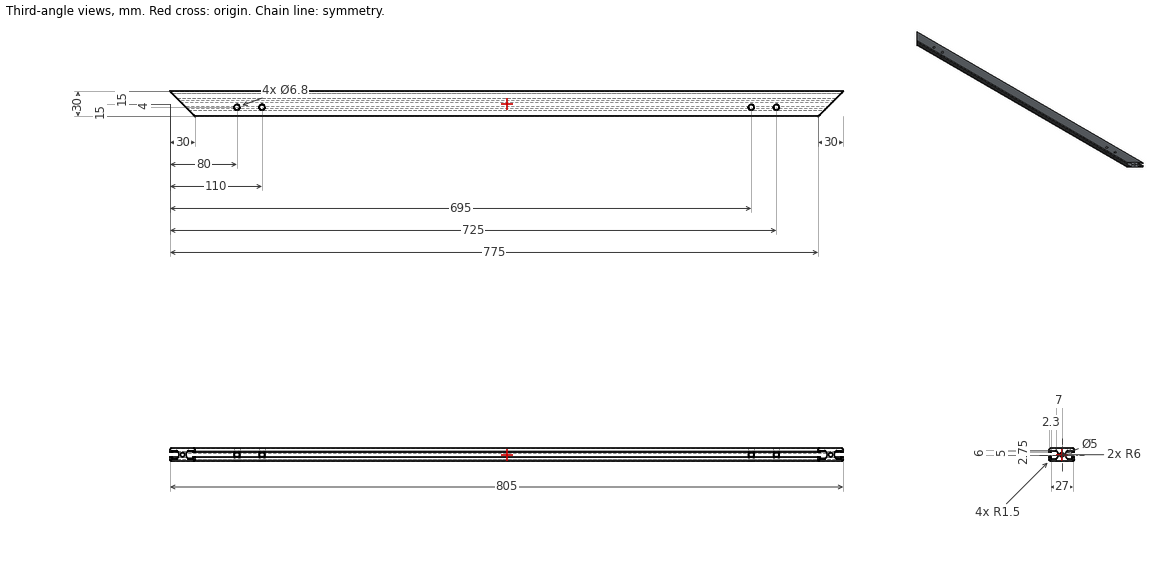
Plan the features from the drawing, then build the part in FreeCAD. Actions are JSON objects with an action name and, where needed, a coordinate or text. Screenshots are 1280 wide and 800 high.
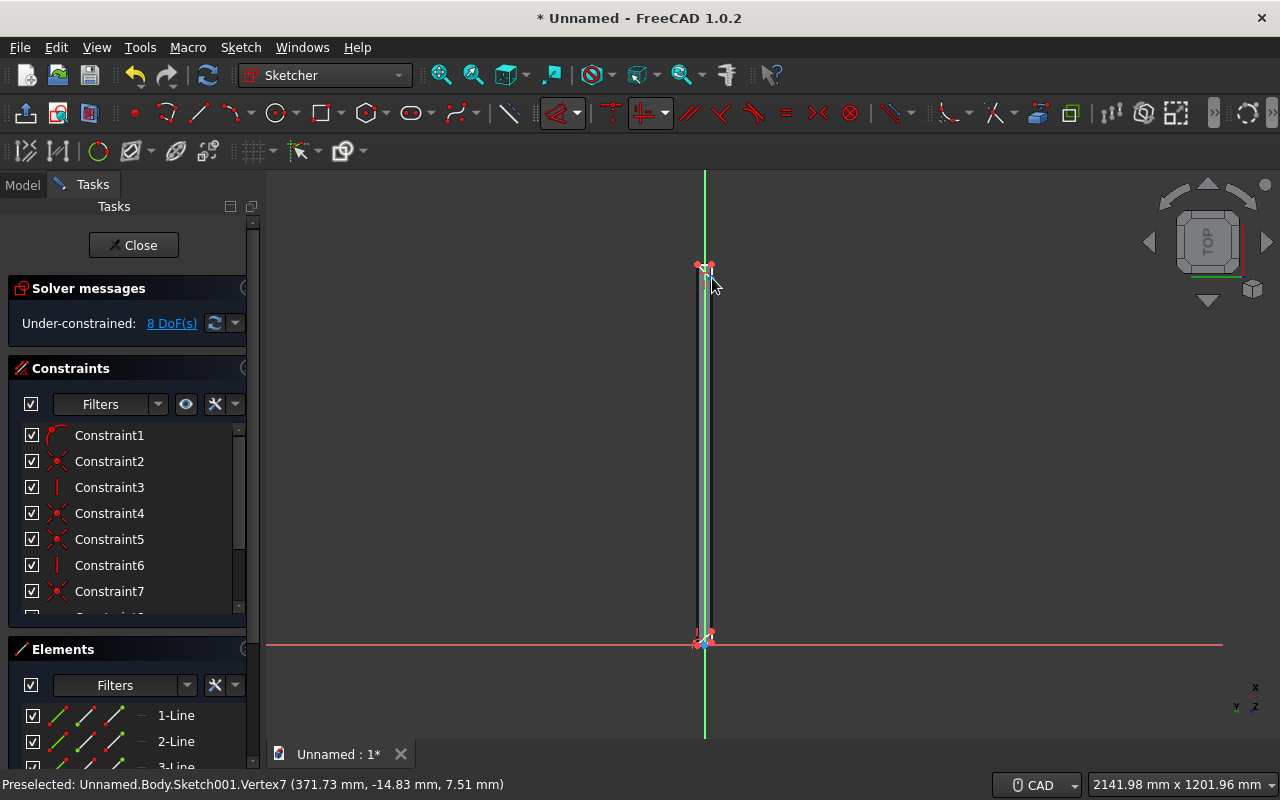
{"action": "scroll", "coordinate": [704, 644], "scroll_direction": "up", "scroll_amount": 7}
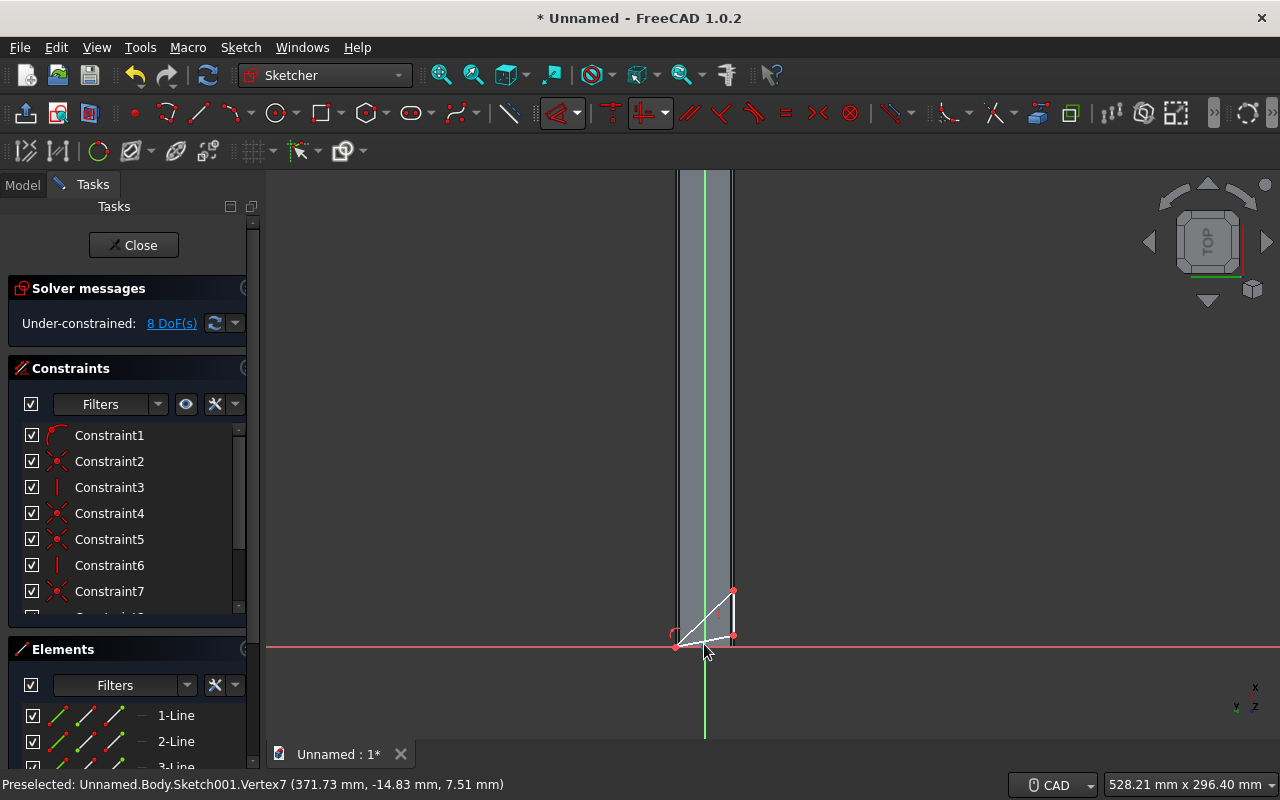
{"action": "left_click", "coordinate": [704, 641]}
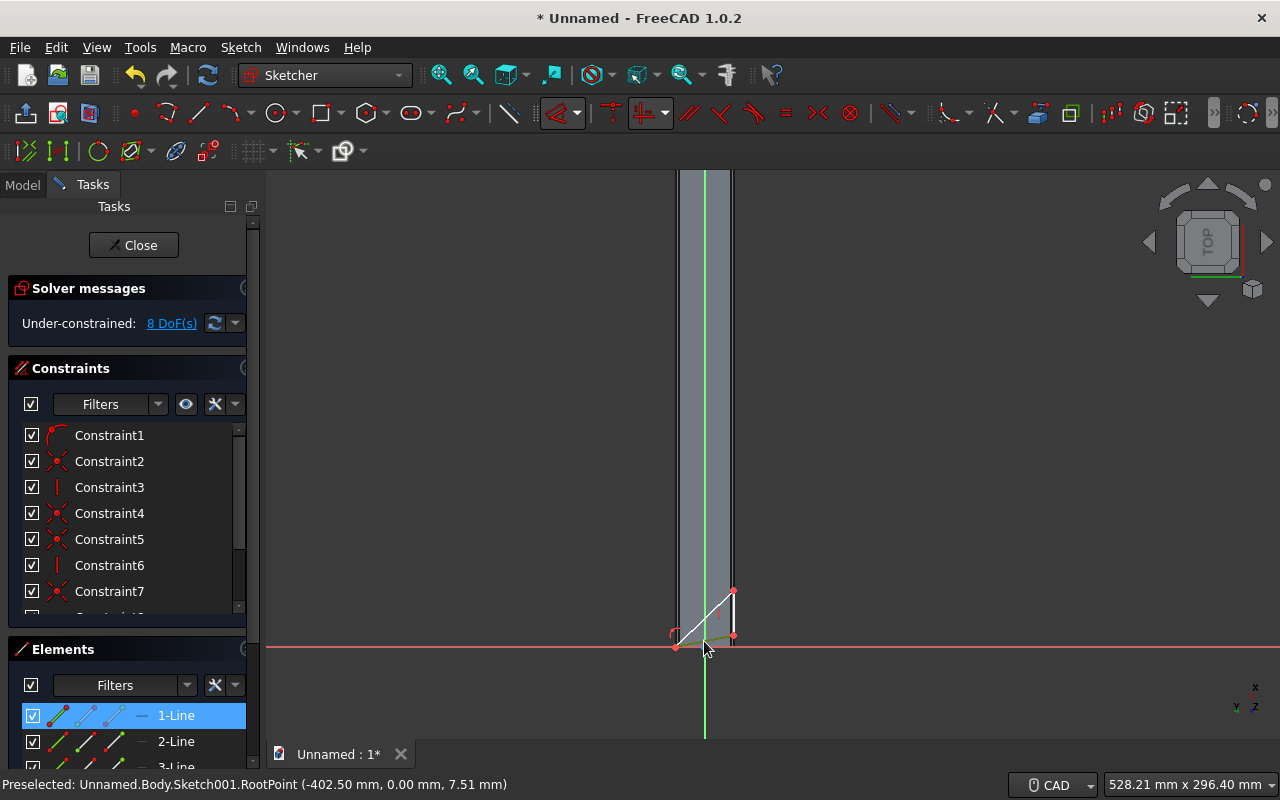
{"action": "key", "text": "h"}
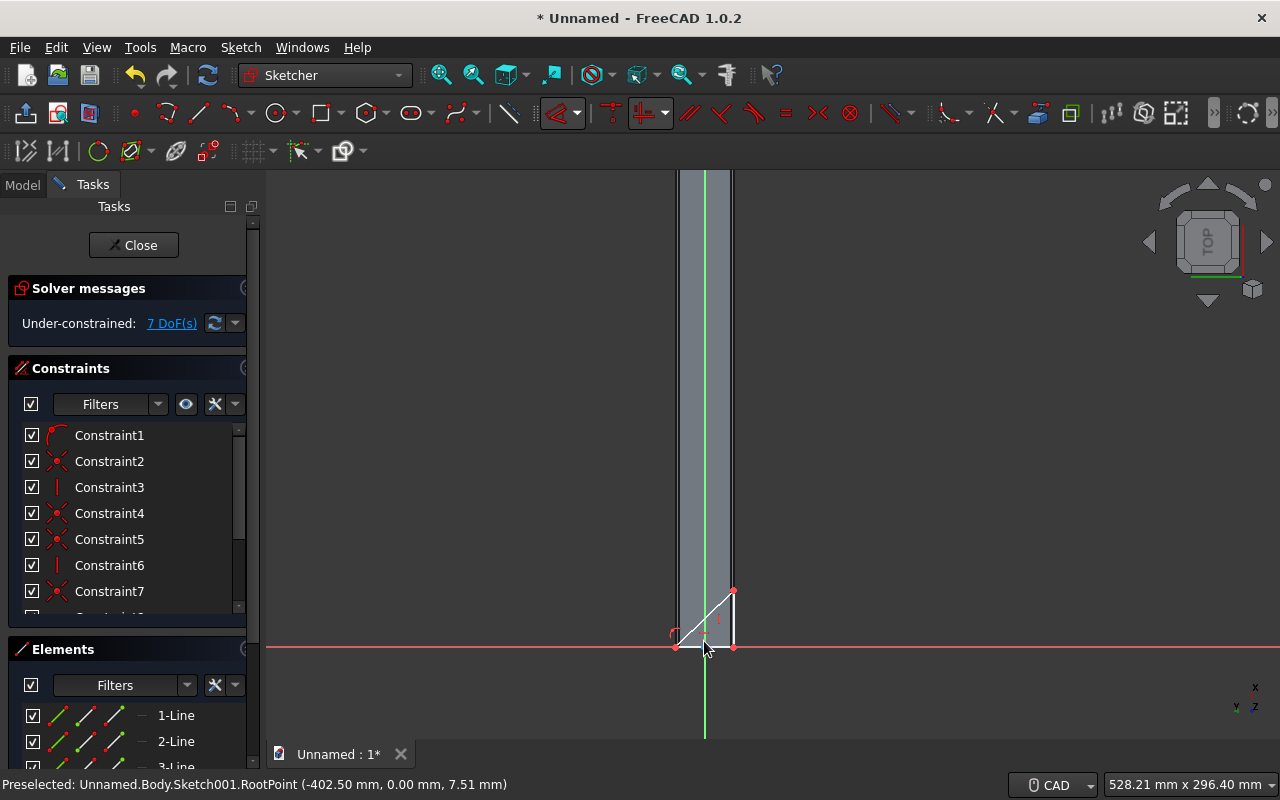
{"action": "left_click", "coordinate": [693, 647]}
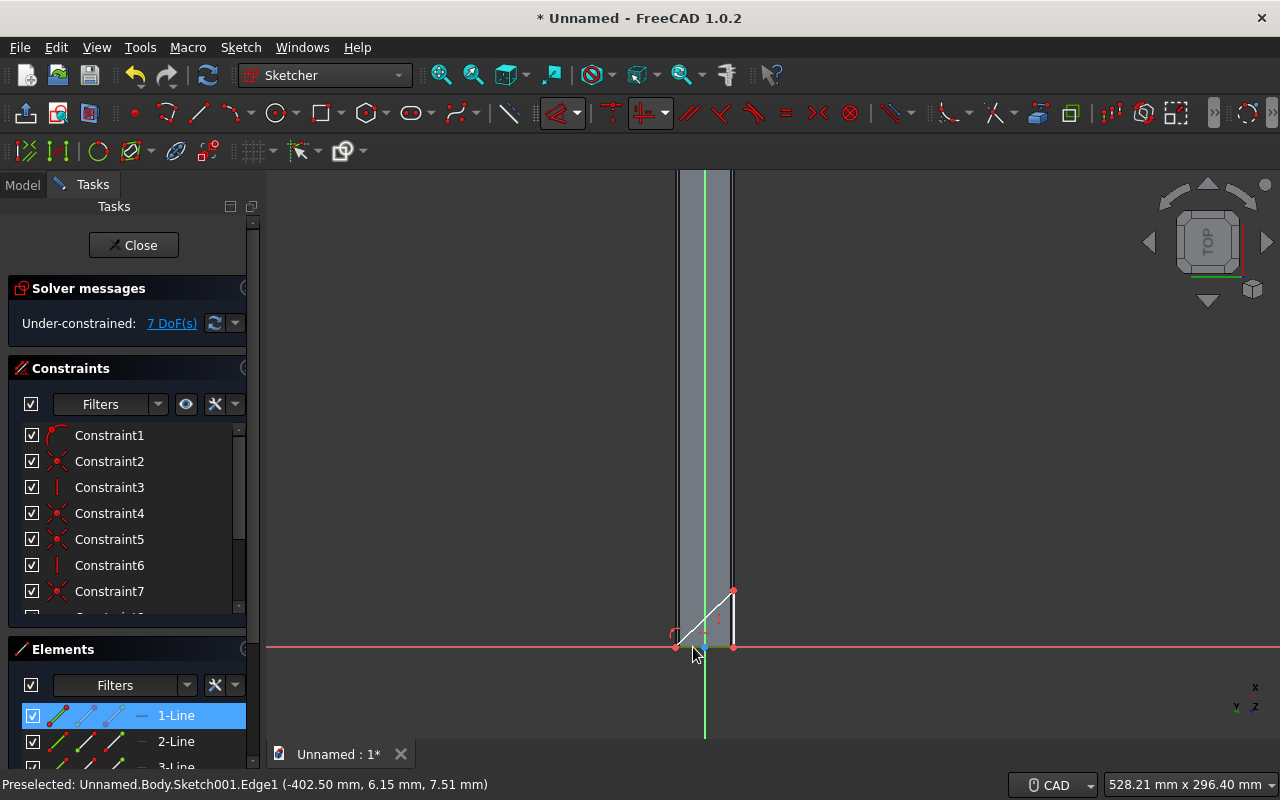
{"action": "key", "text": "l"}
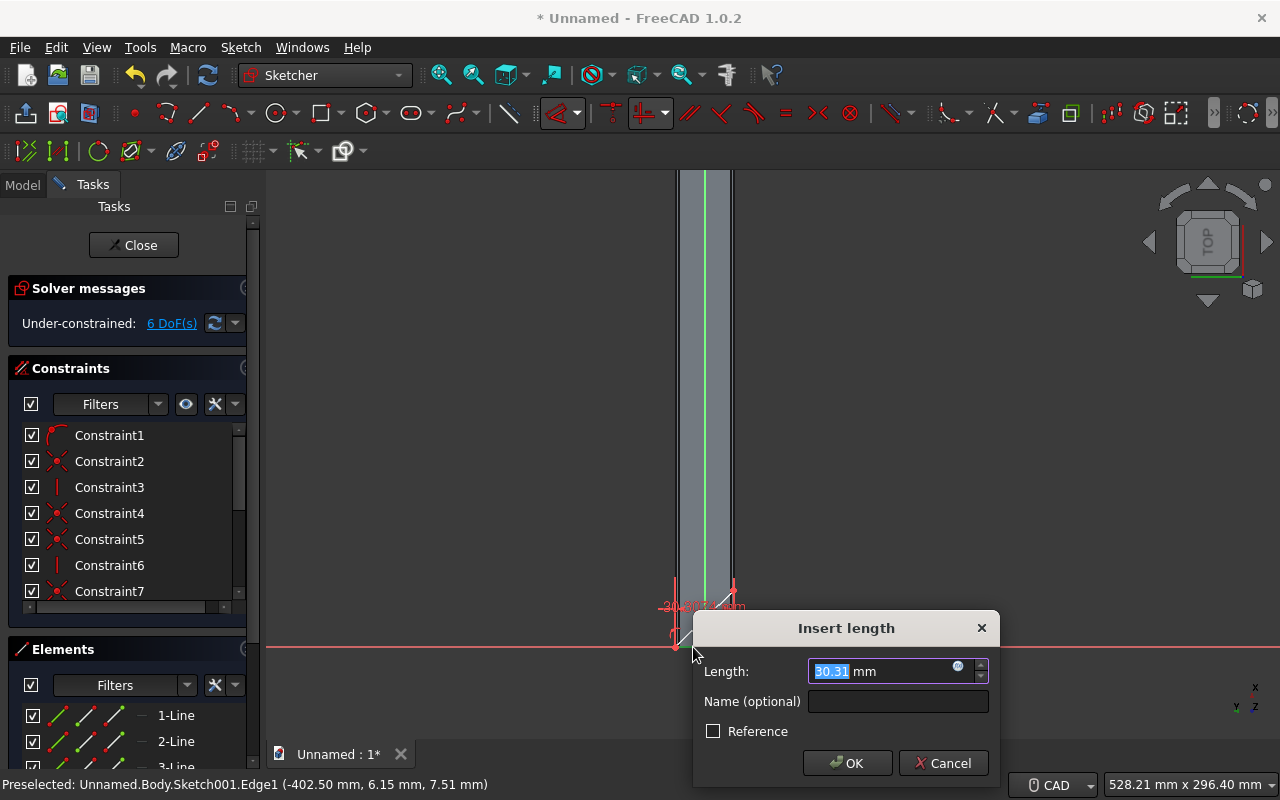
{"action": "type", "text": "30"}
{"action": "key", "text": "Return"}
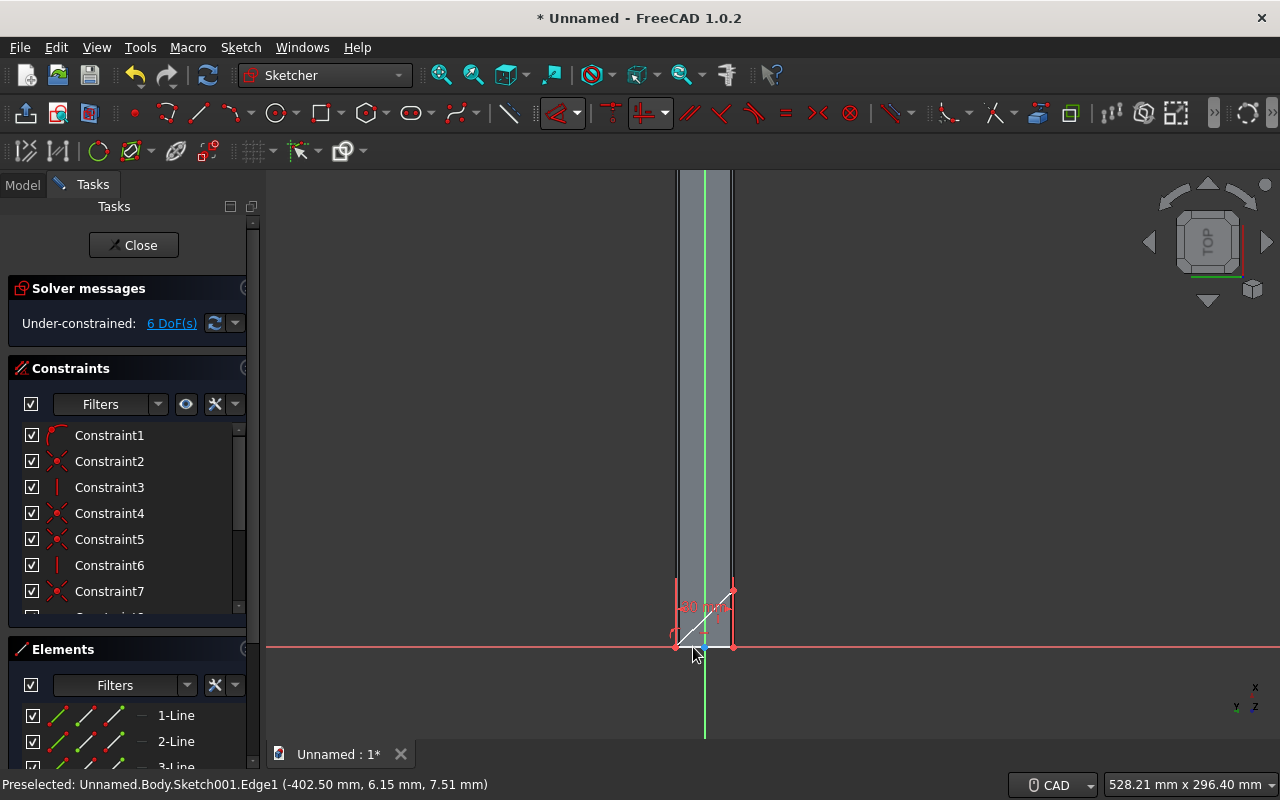
{"action": "left_click", "coordinate": [733, 630]}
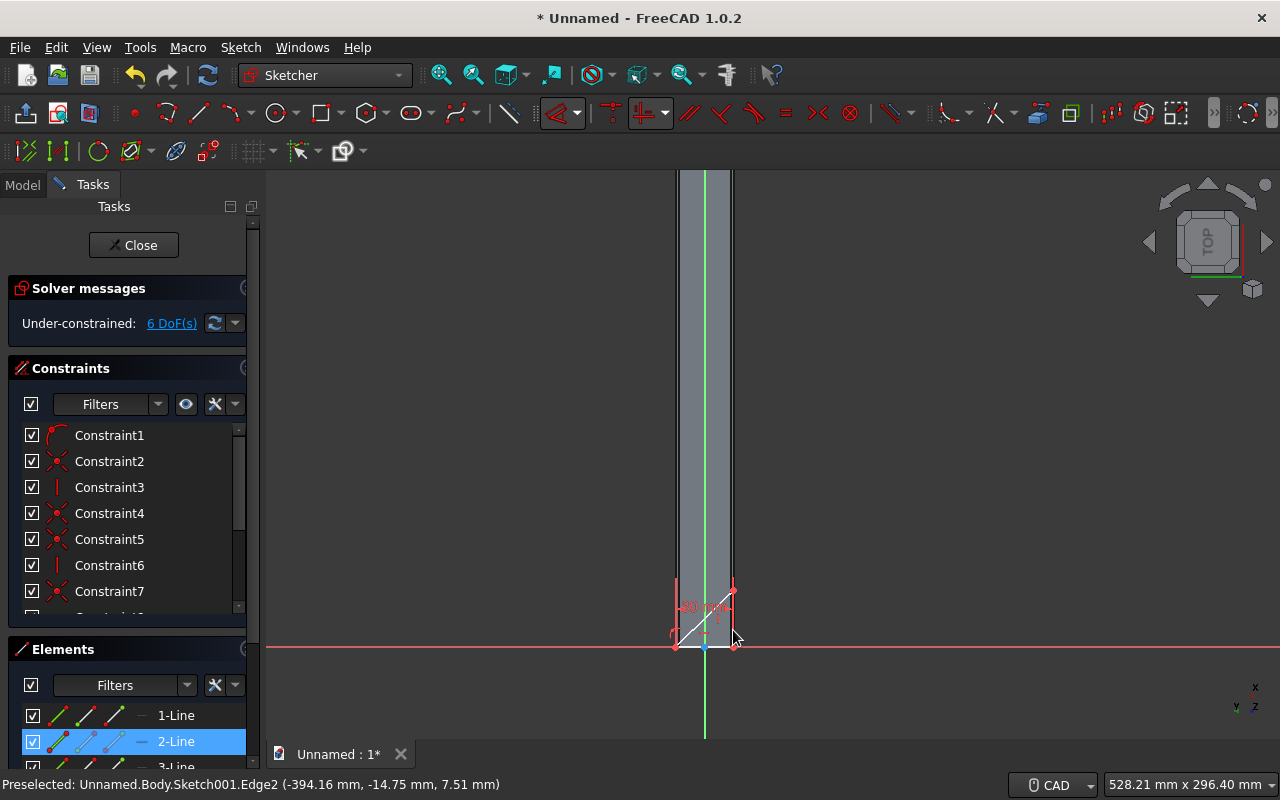
{"action": "key", "text": "i"}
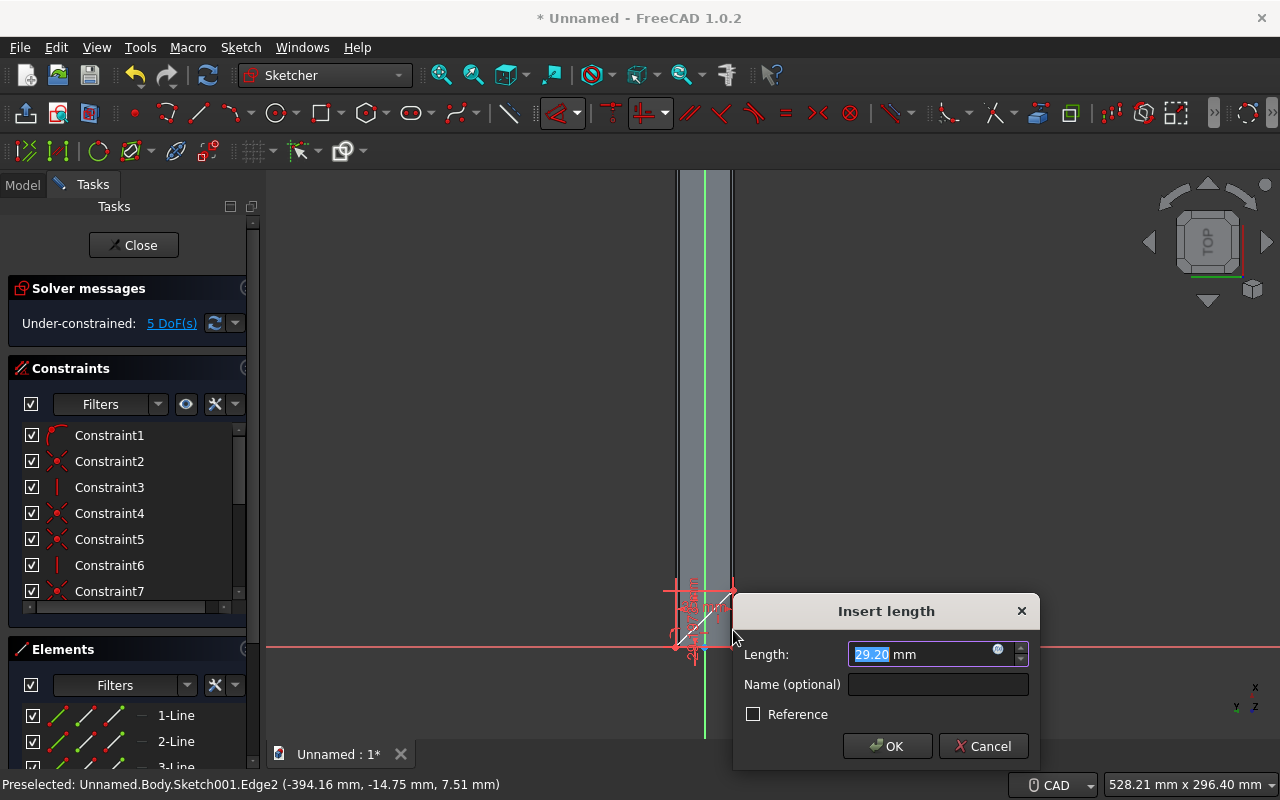
{"action": "type", "text": "30"}
{"action": "key", "text": "Return"}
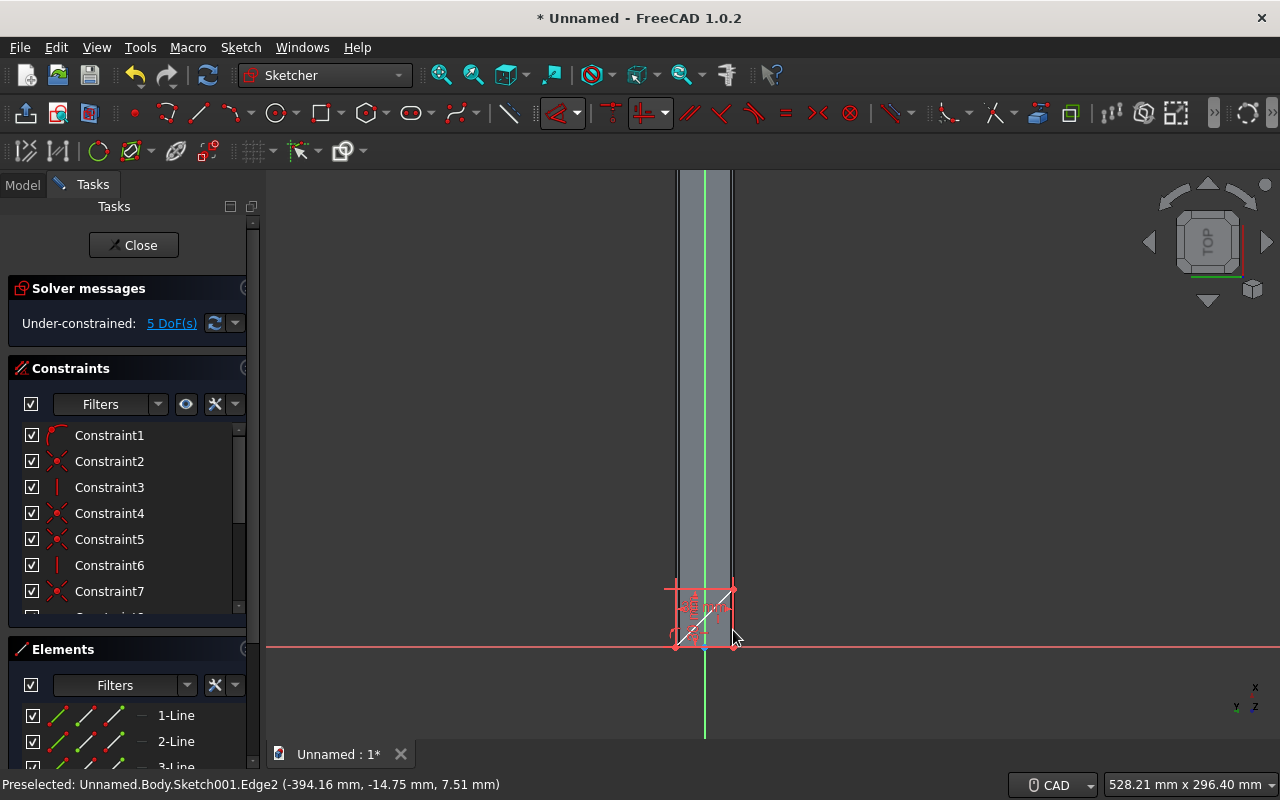
{"action": "scroll", "coordinate": [704, 644], "scroll_direction": "down", "scroll_amount": 7}